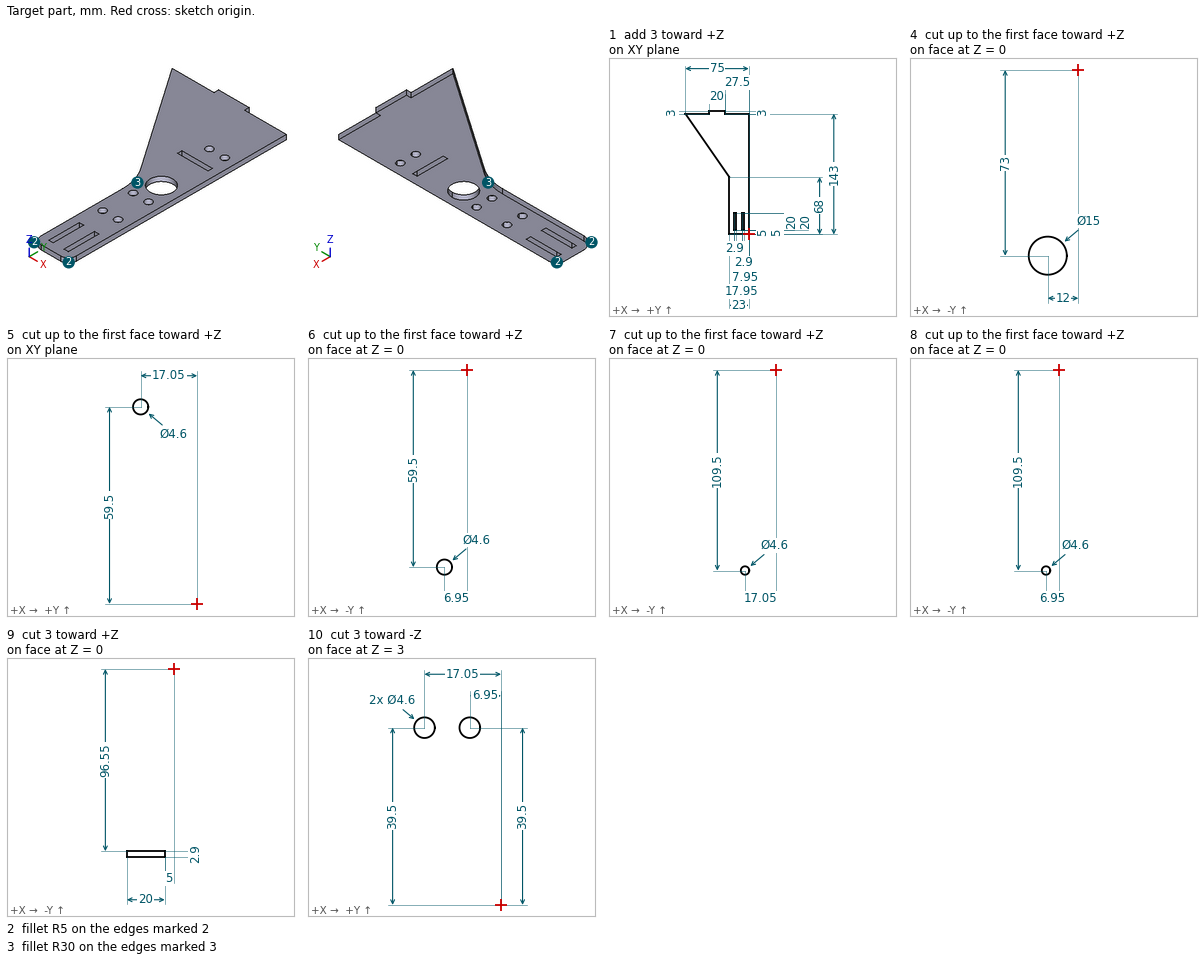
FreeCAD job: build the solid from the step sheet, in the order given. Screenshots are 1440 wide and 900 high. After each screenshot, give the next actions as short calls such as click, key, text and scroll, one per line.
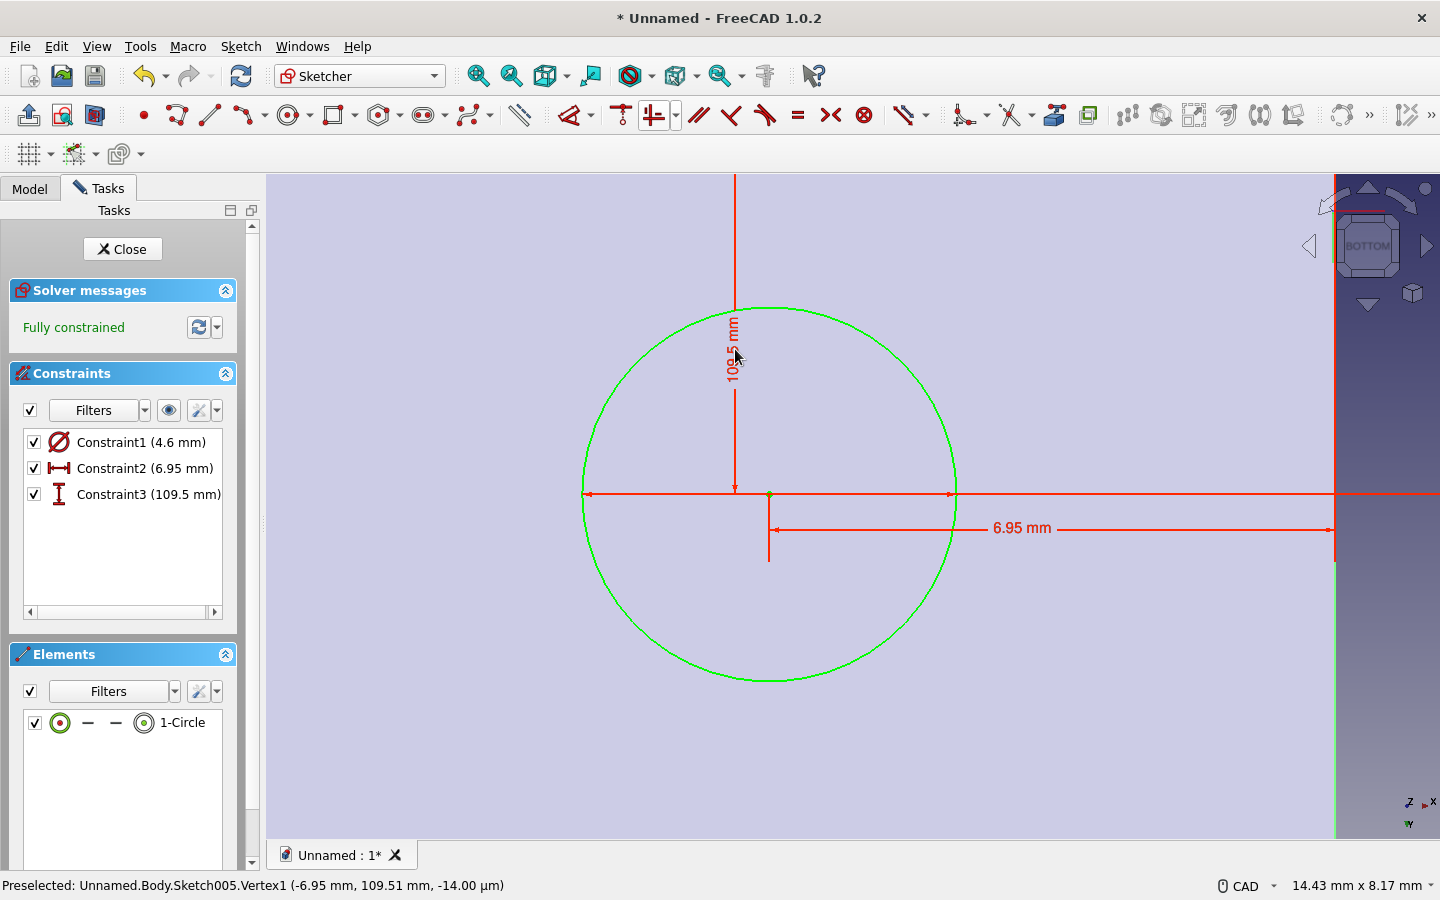
click(123, 249)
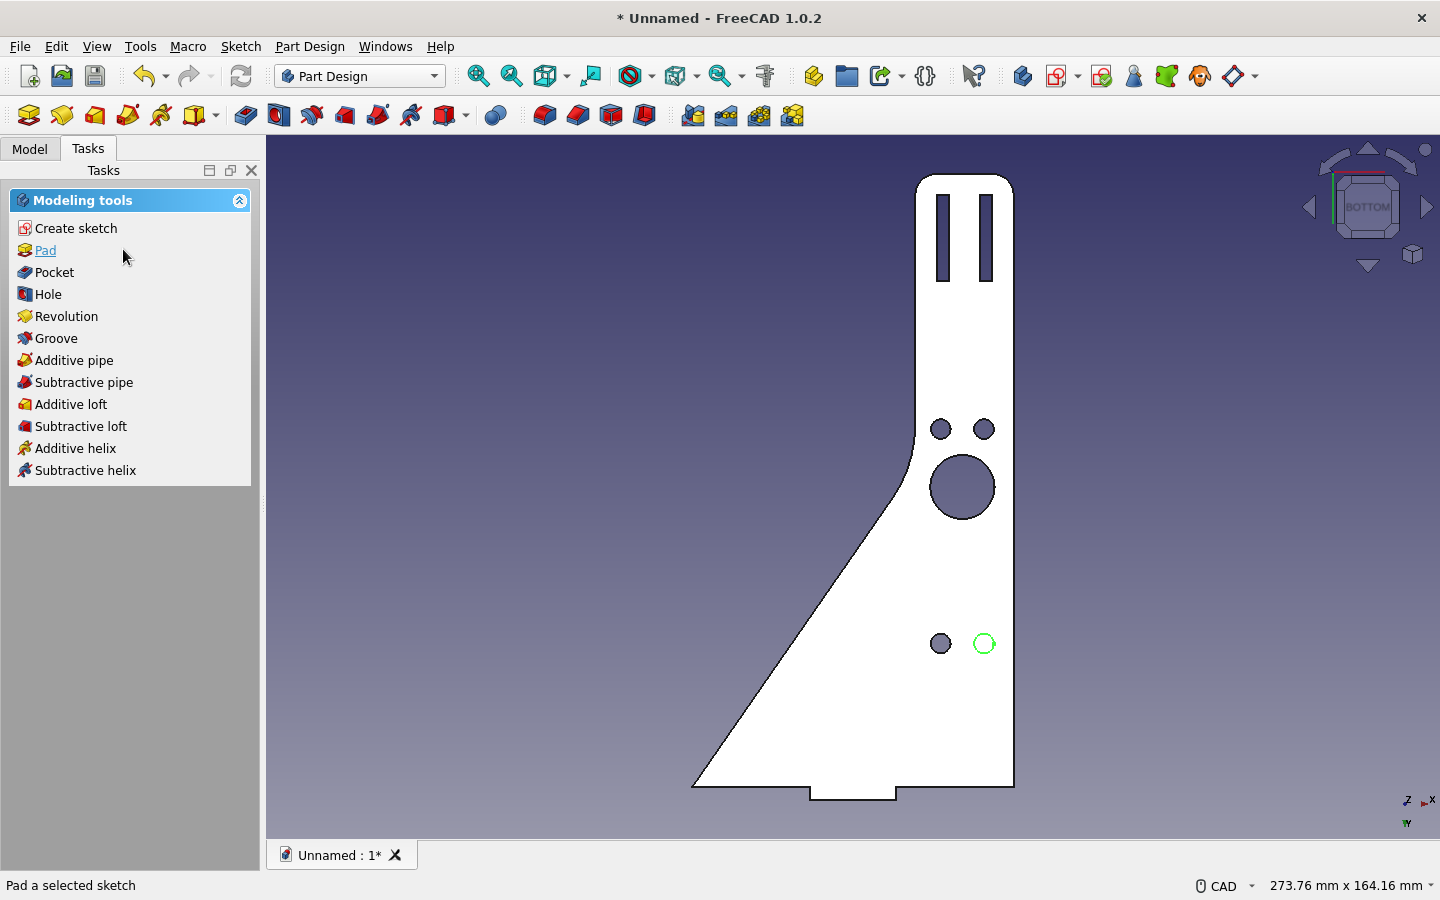
click(246, 116)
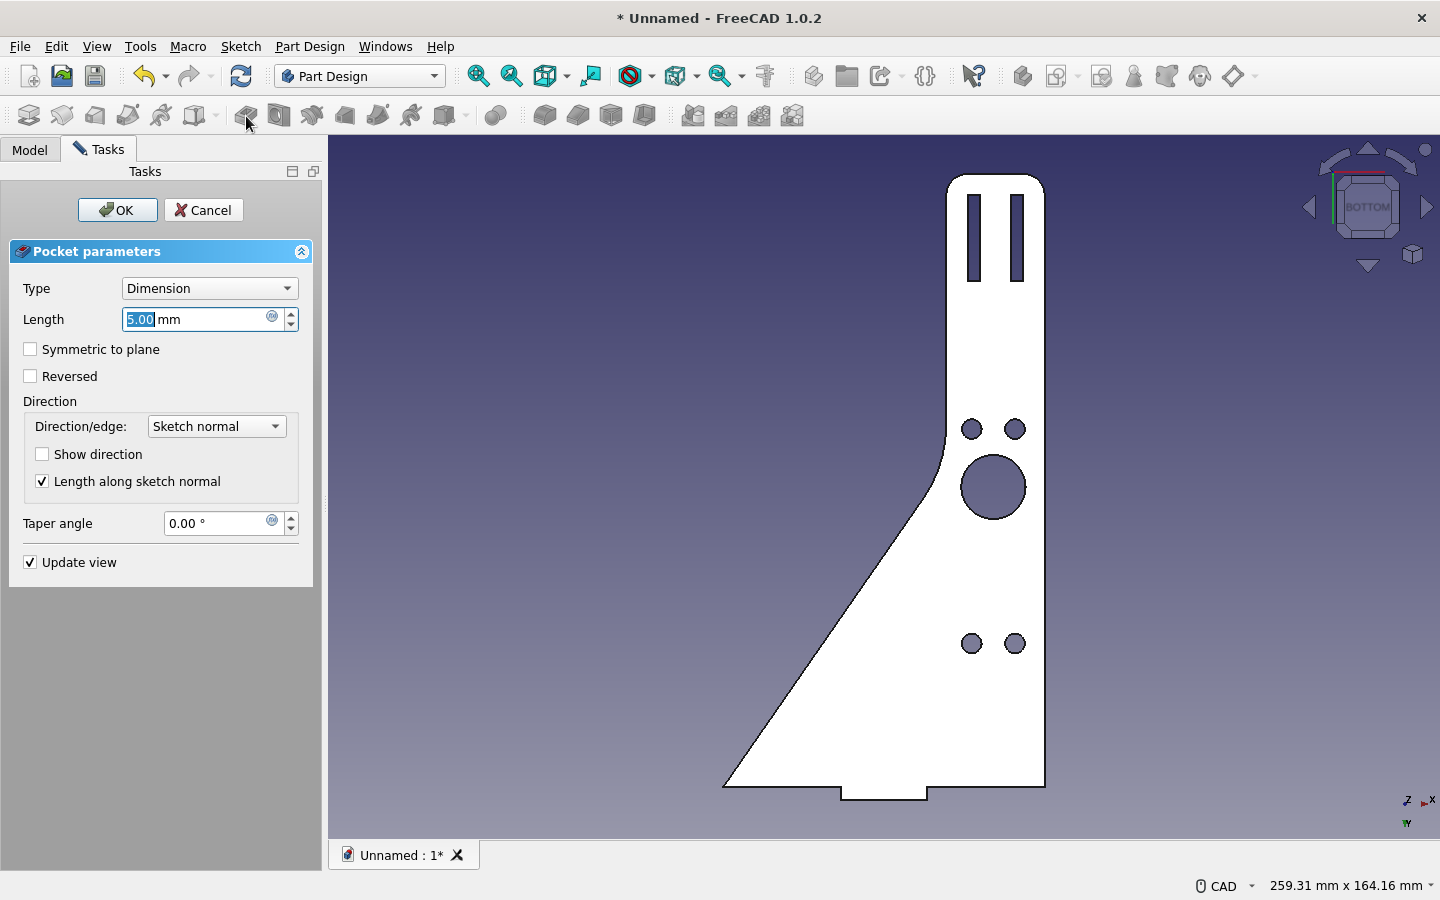
click(210, 288)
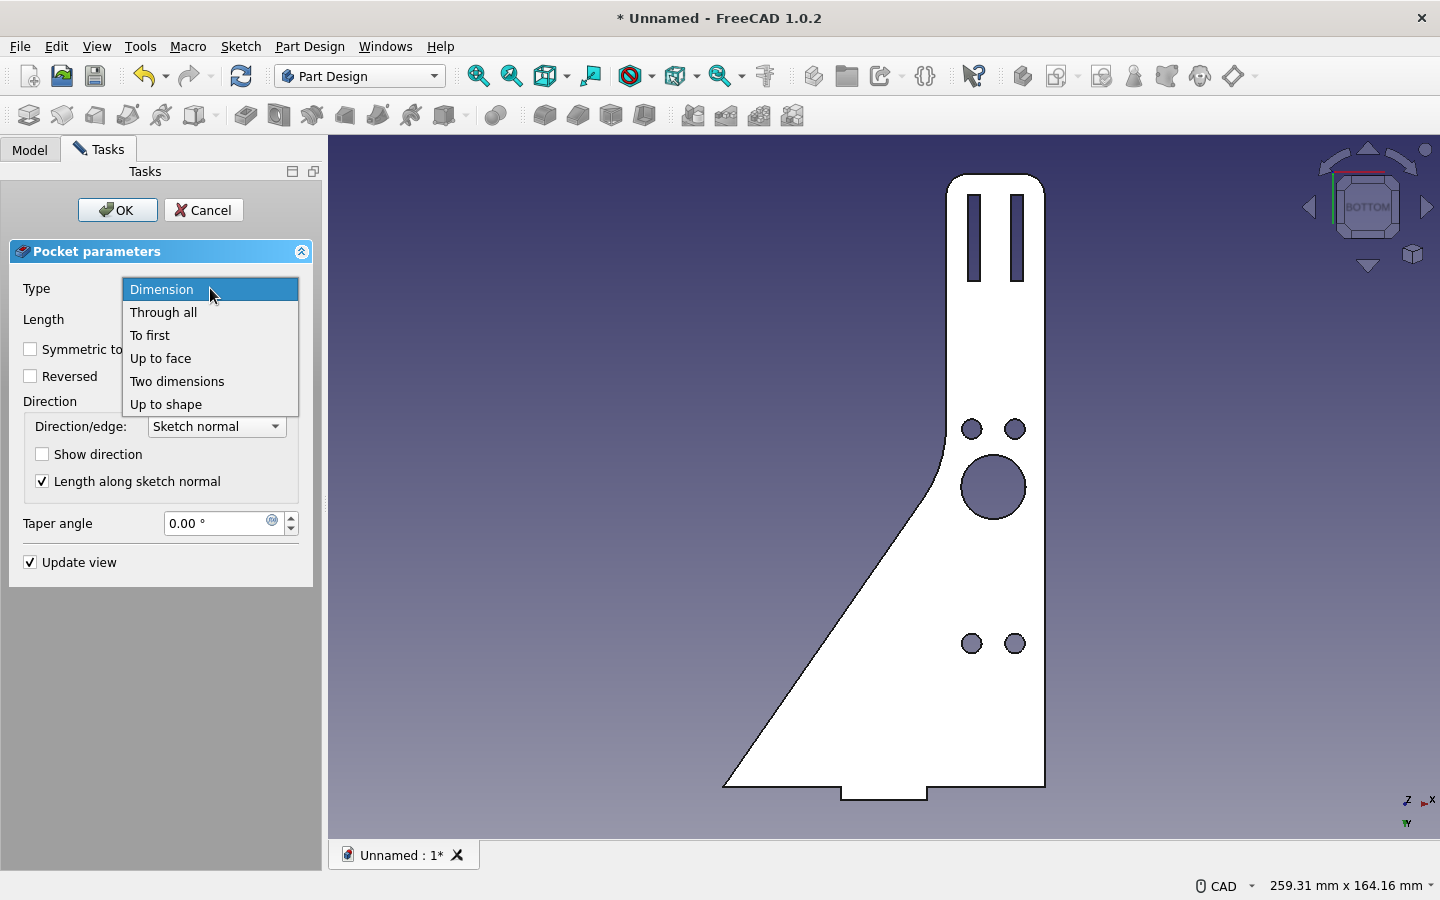
click(208, 336)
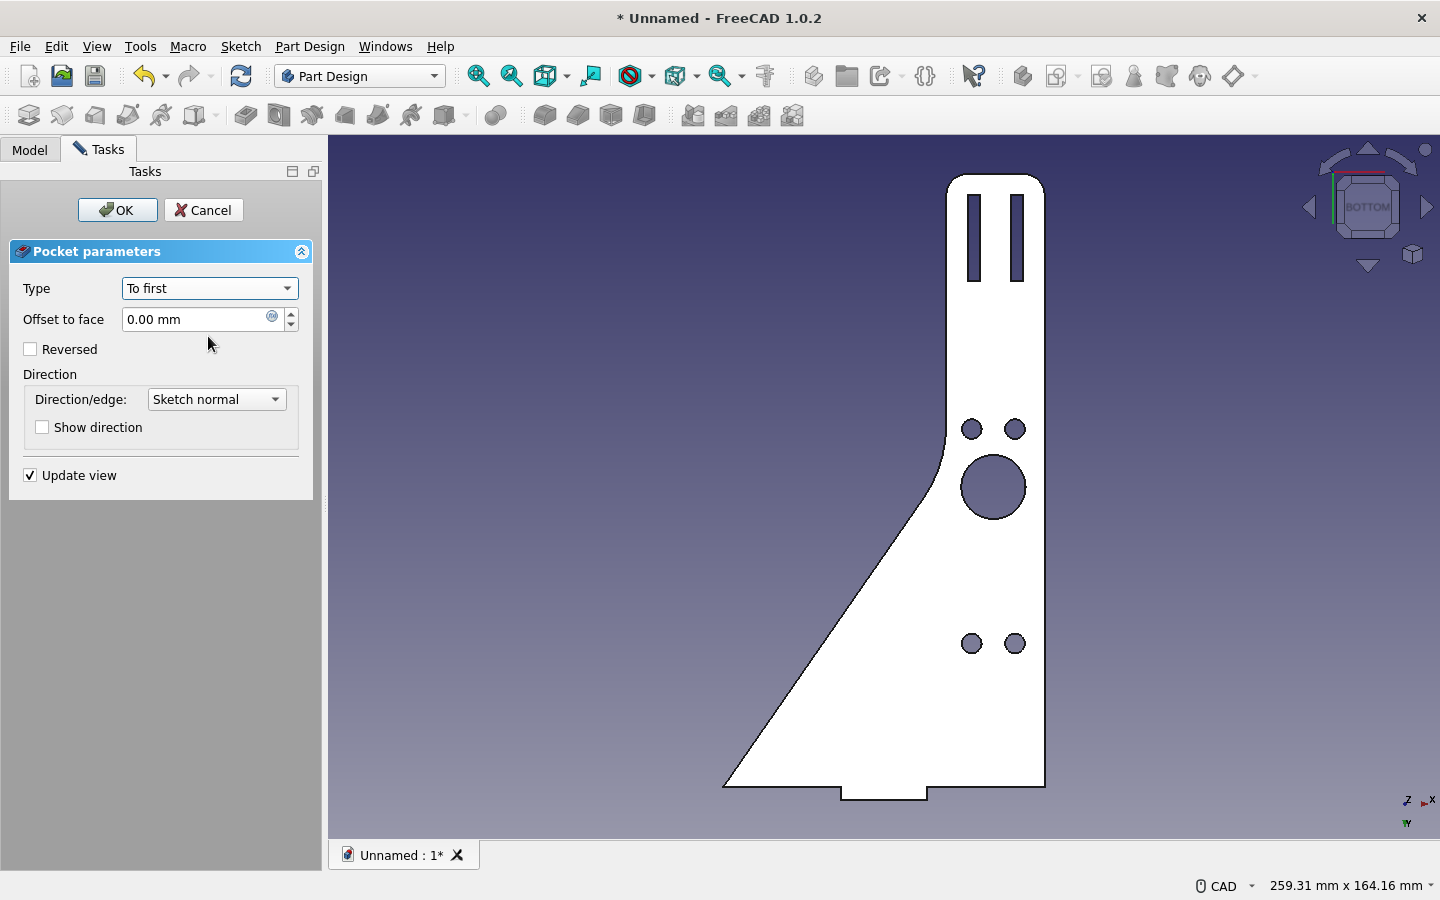
click(118, 210)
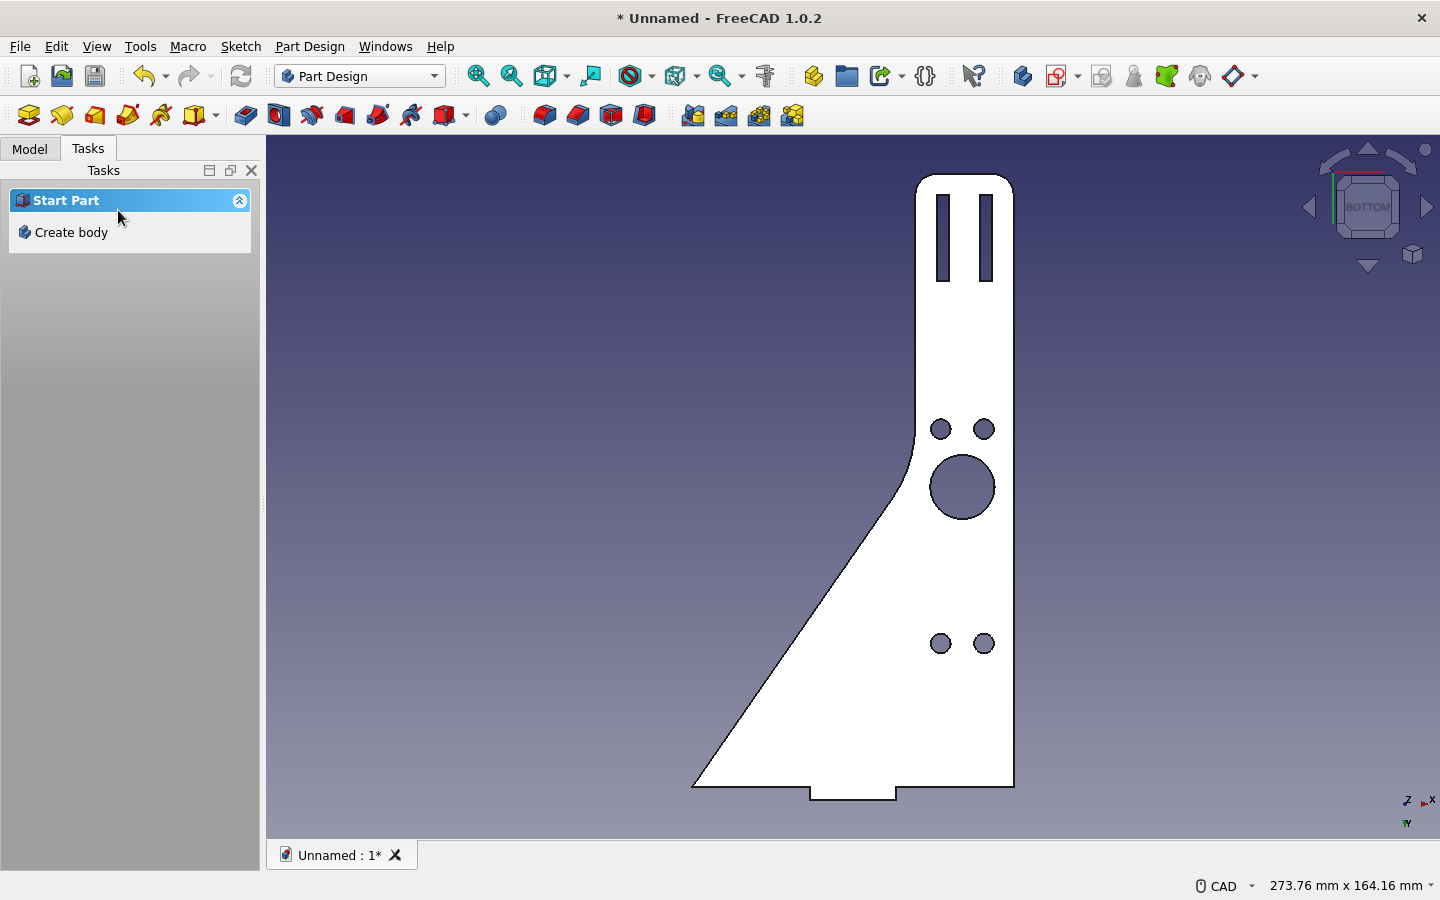
click(853, 665)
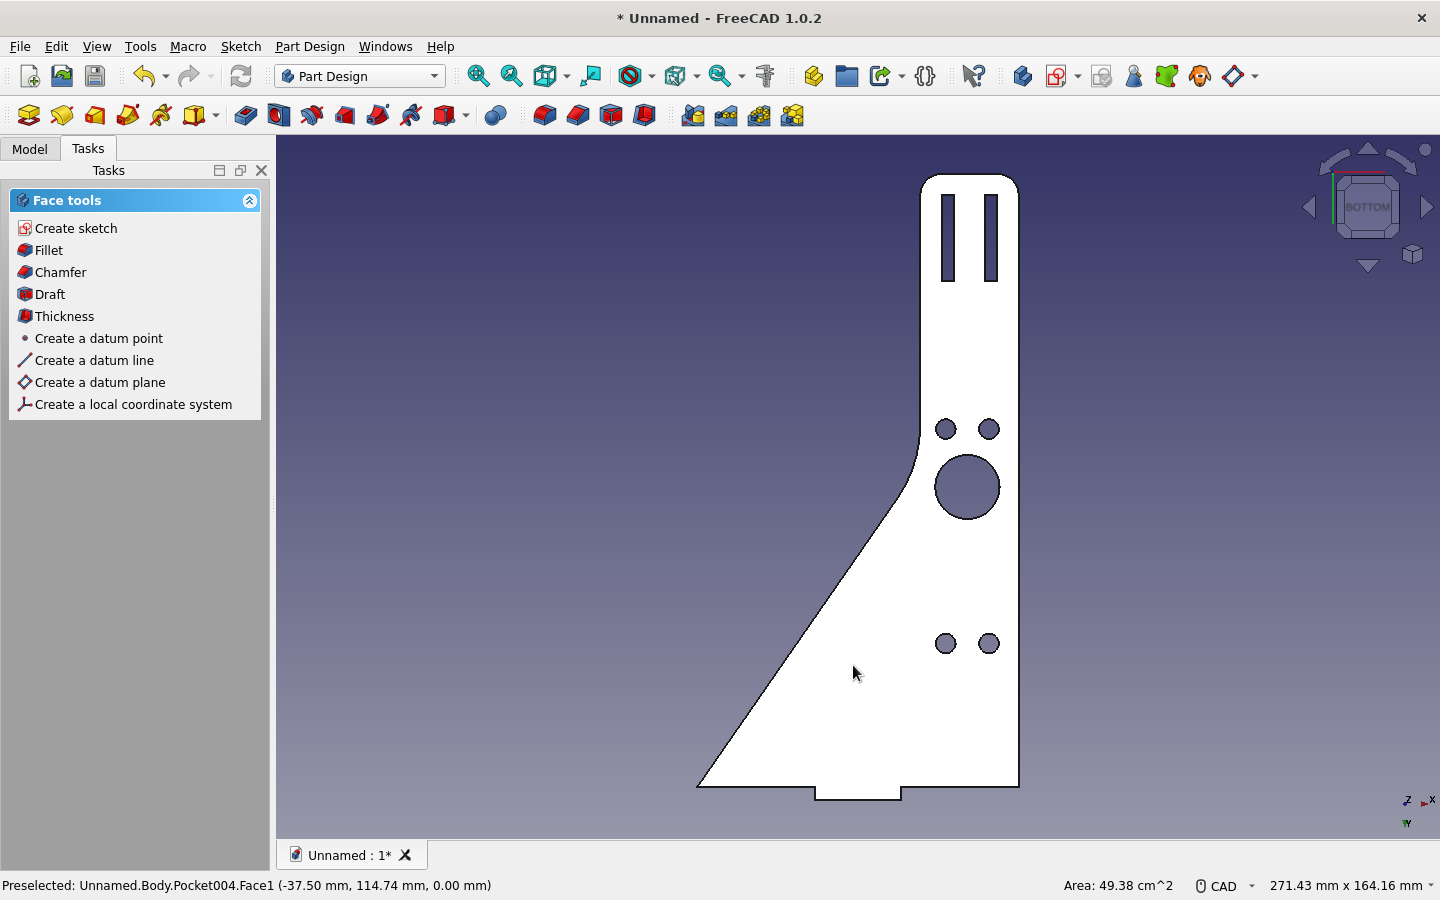
click(1056, 76)